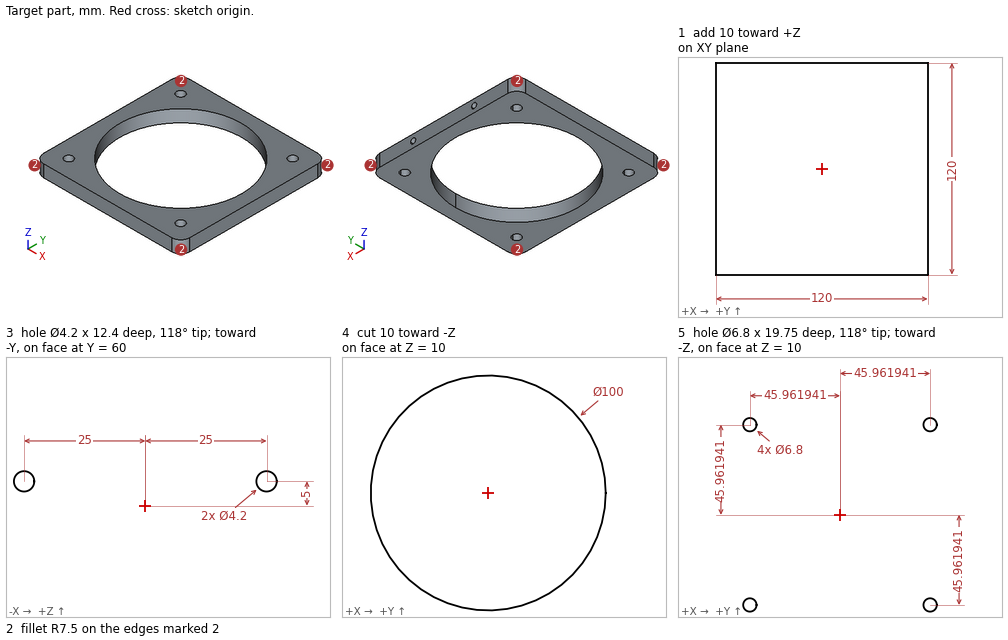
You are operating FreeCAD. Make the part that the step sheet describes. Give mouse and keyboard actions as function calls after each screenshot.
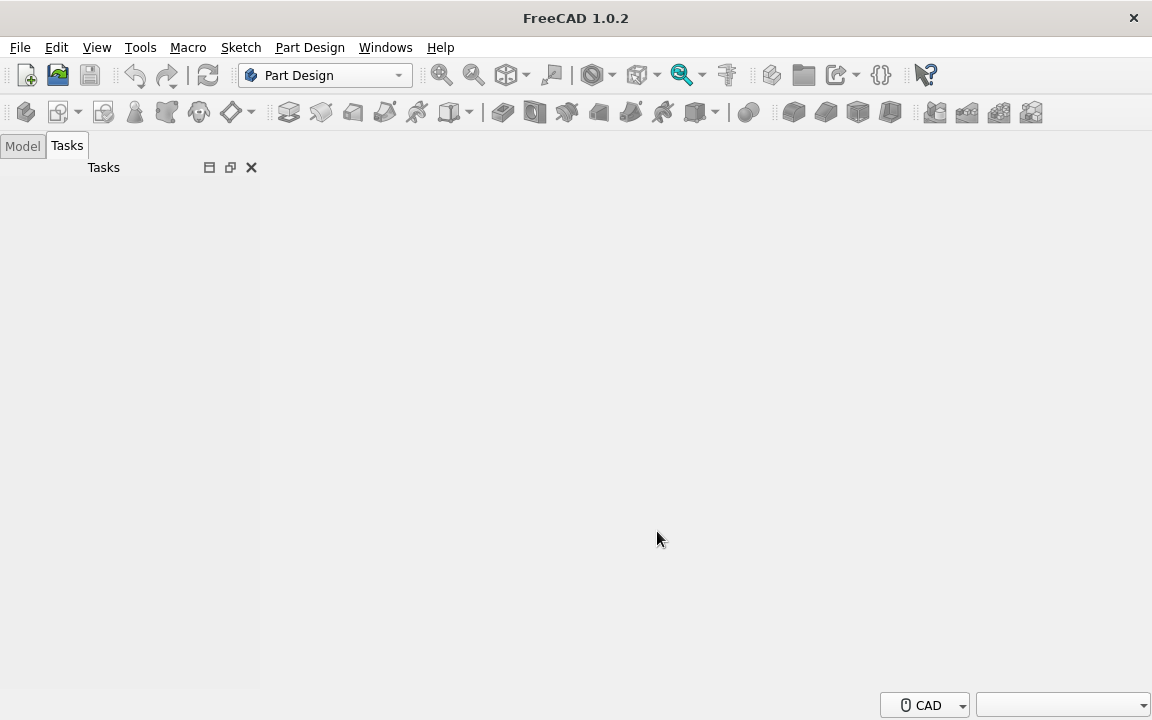
click(26, 76)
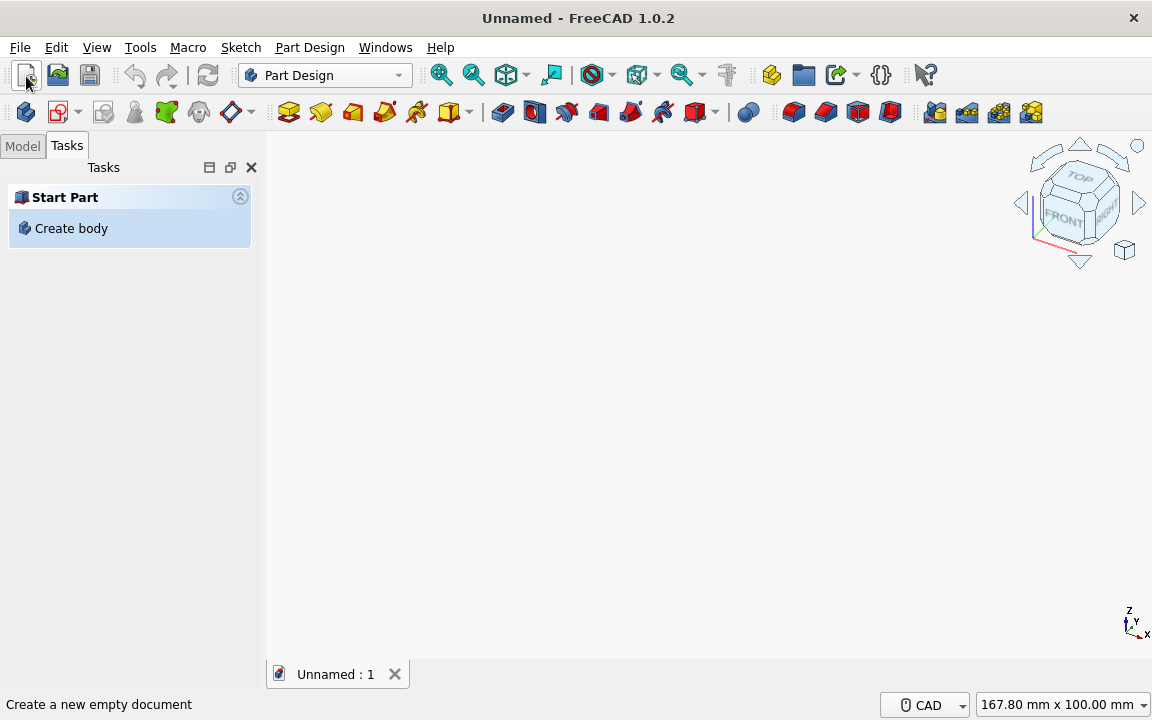
click(58, 112)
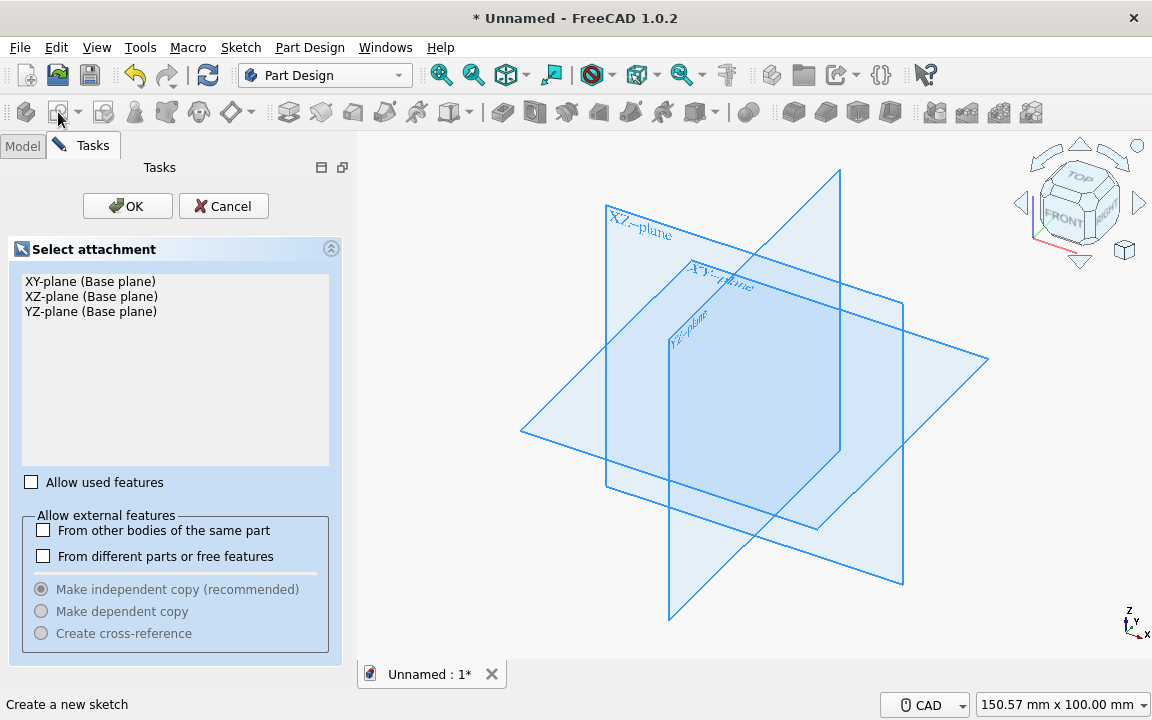
click(82, 282)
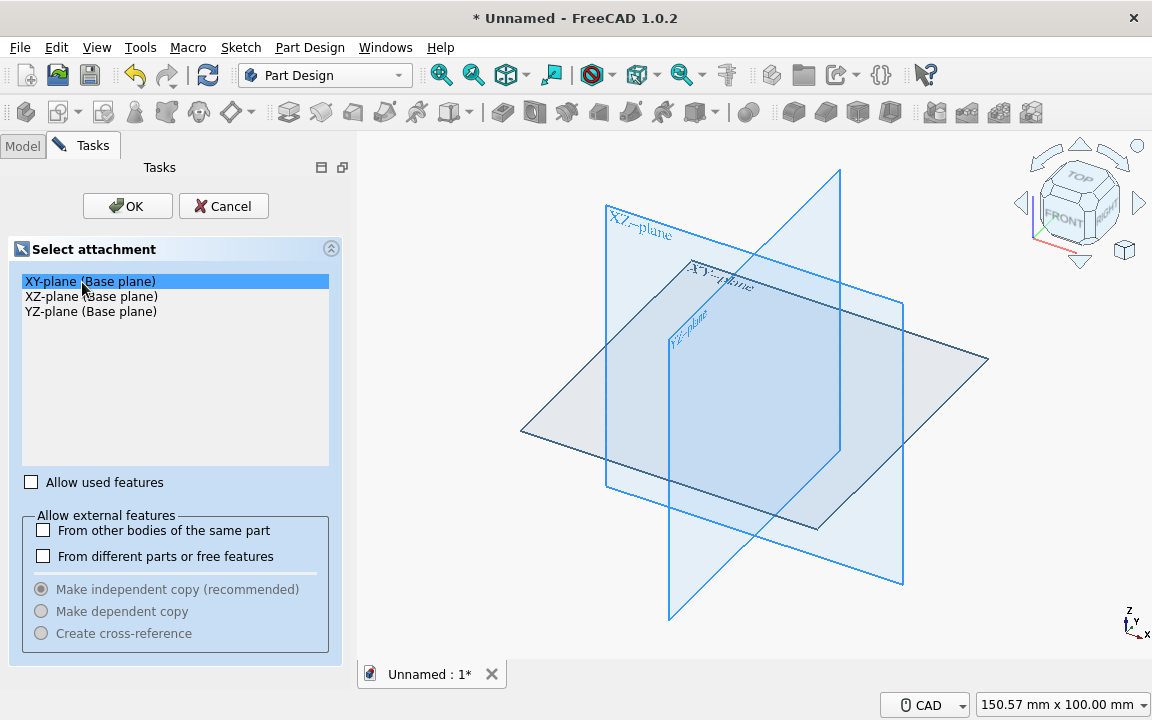
click(128, 206)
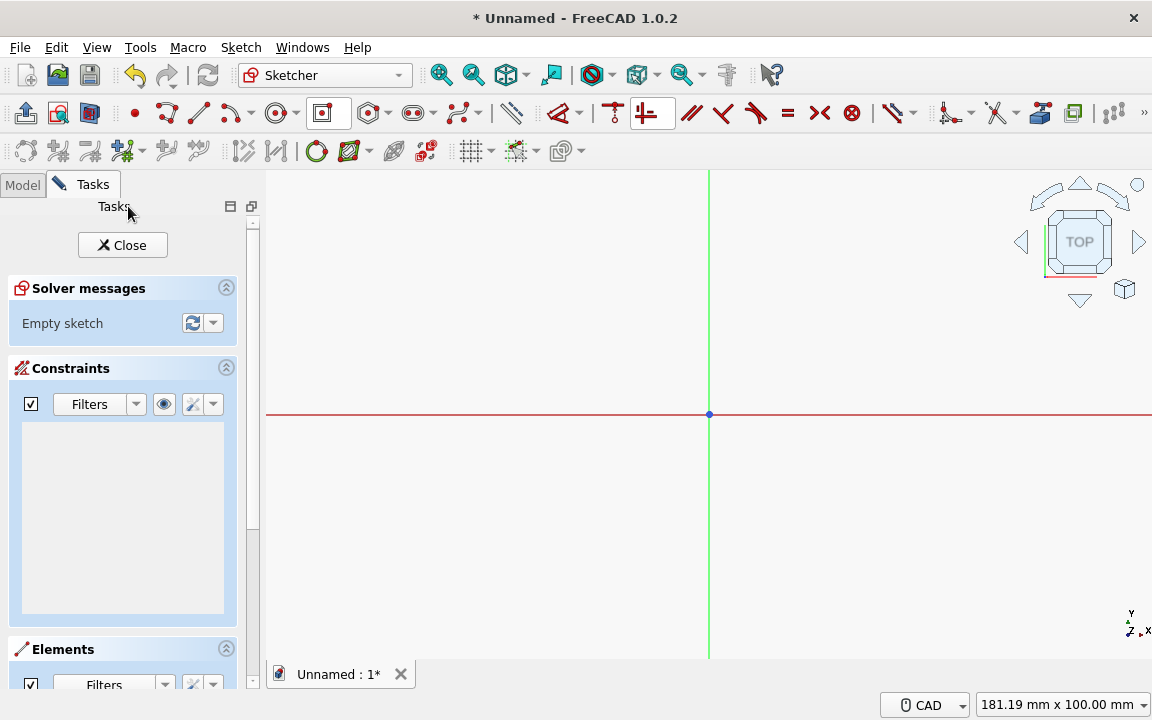
scroll(557, 414, down, 3)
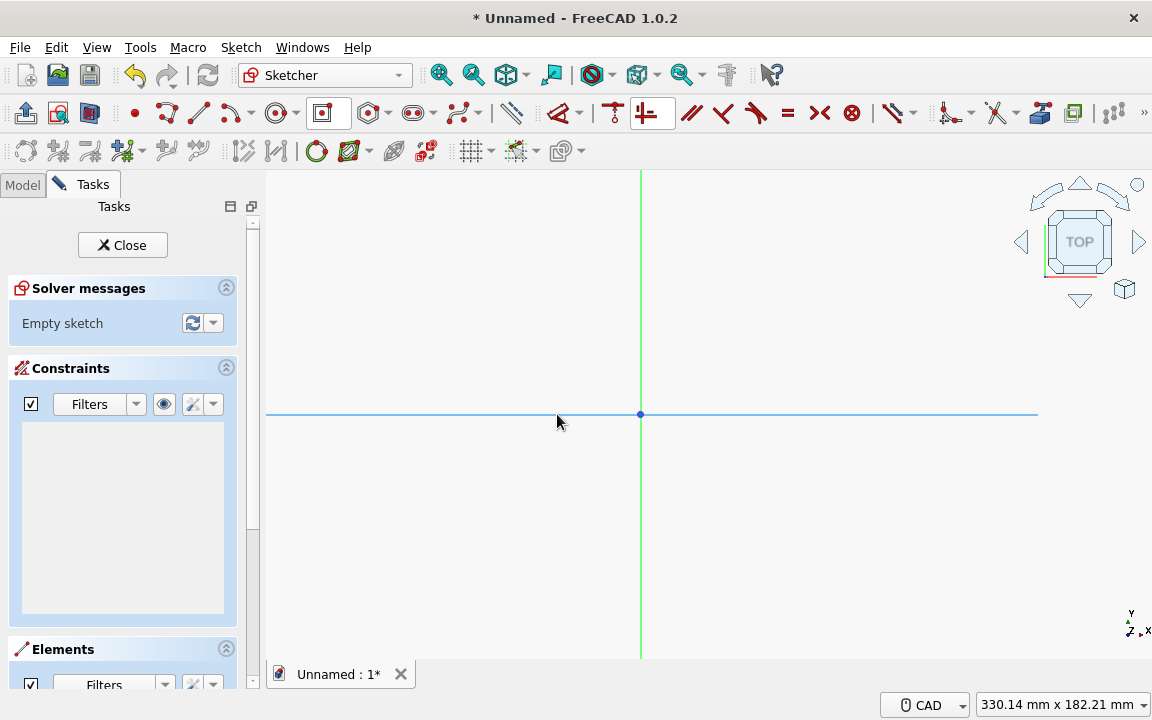
click(322, 114)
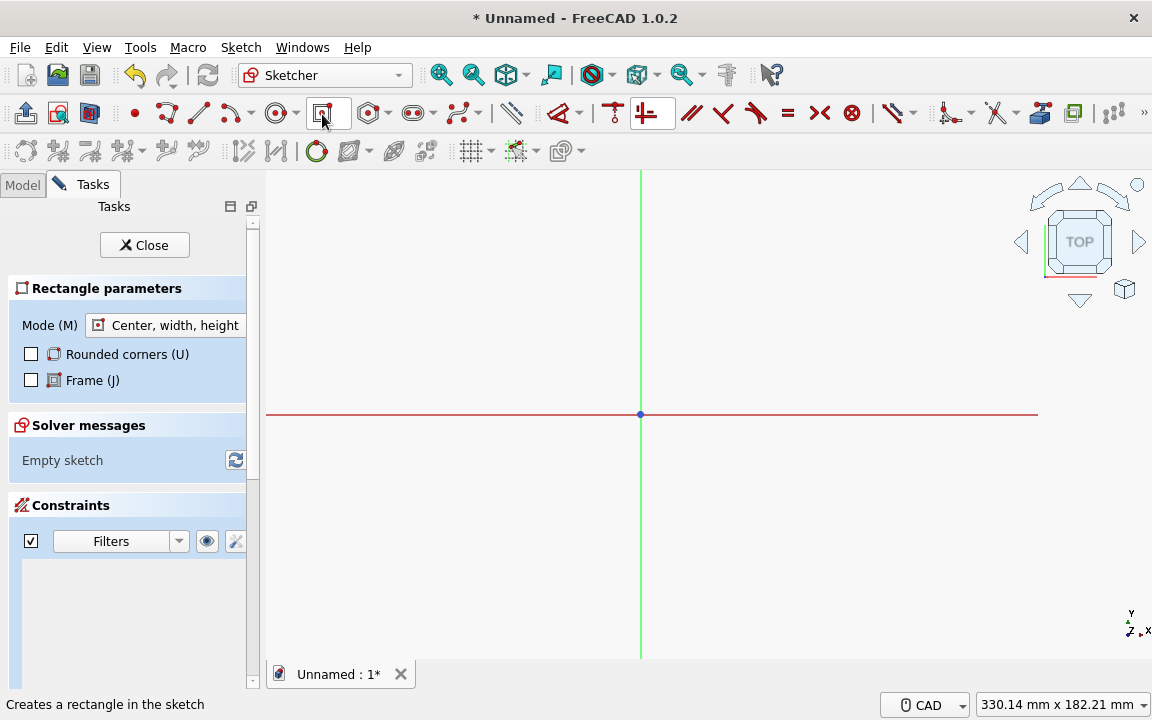
click(641, 414)
click(802, 253)
key(Escape)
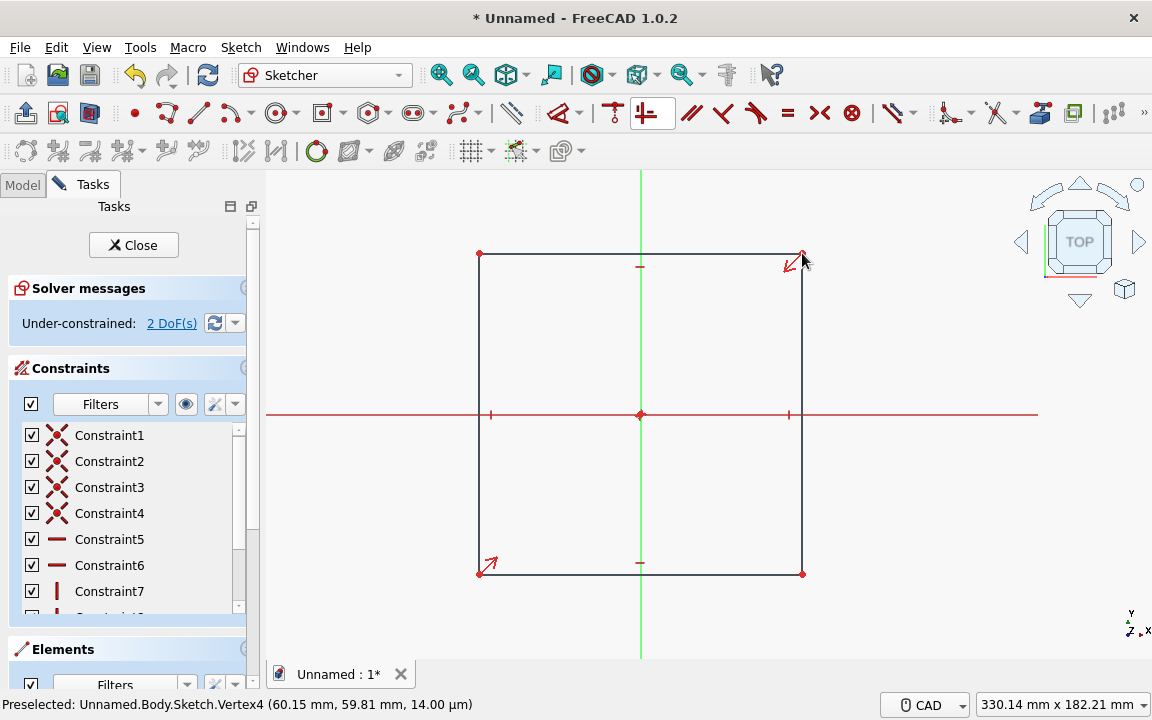
click(558, 114)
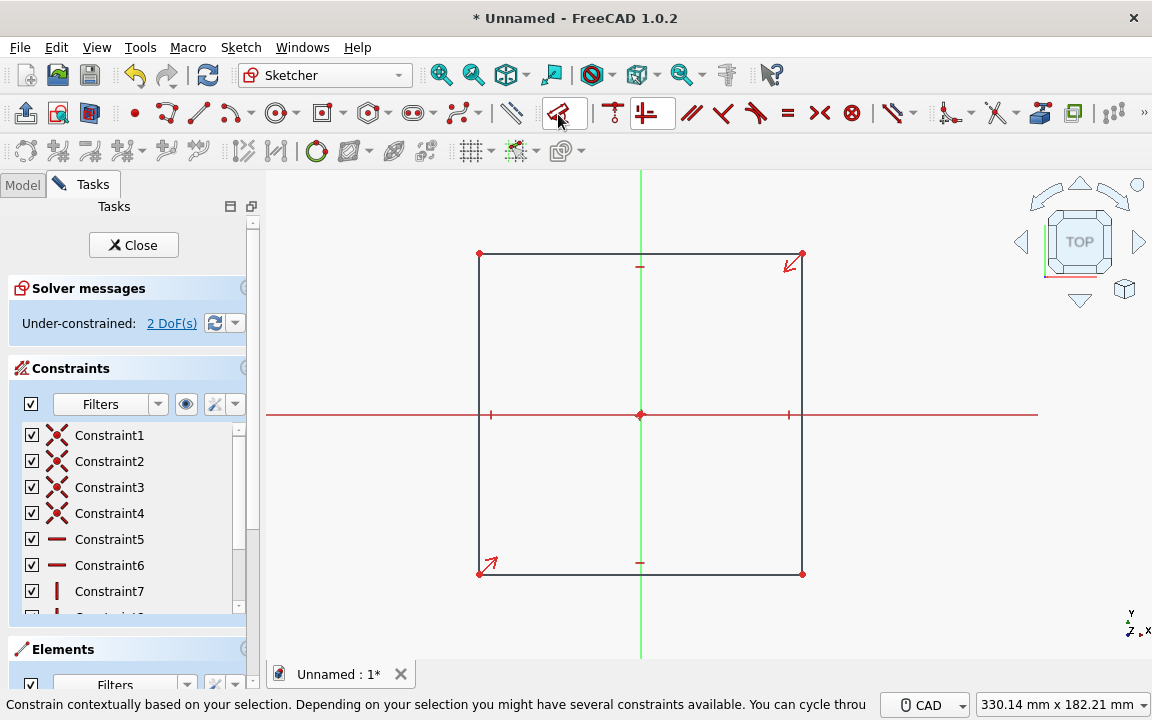
click(576, 575)
click(566, 609)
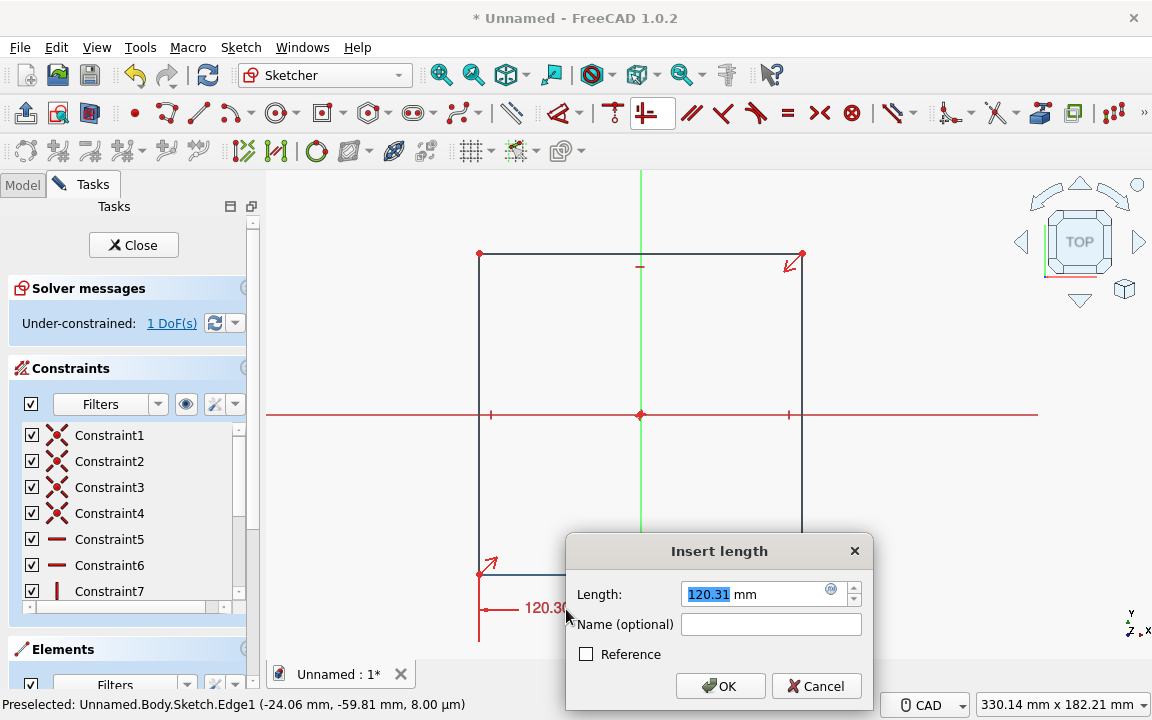
text(120)
key(Return)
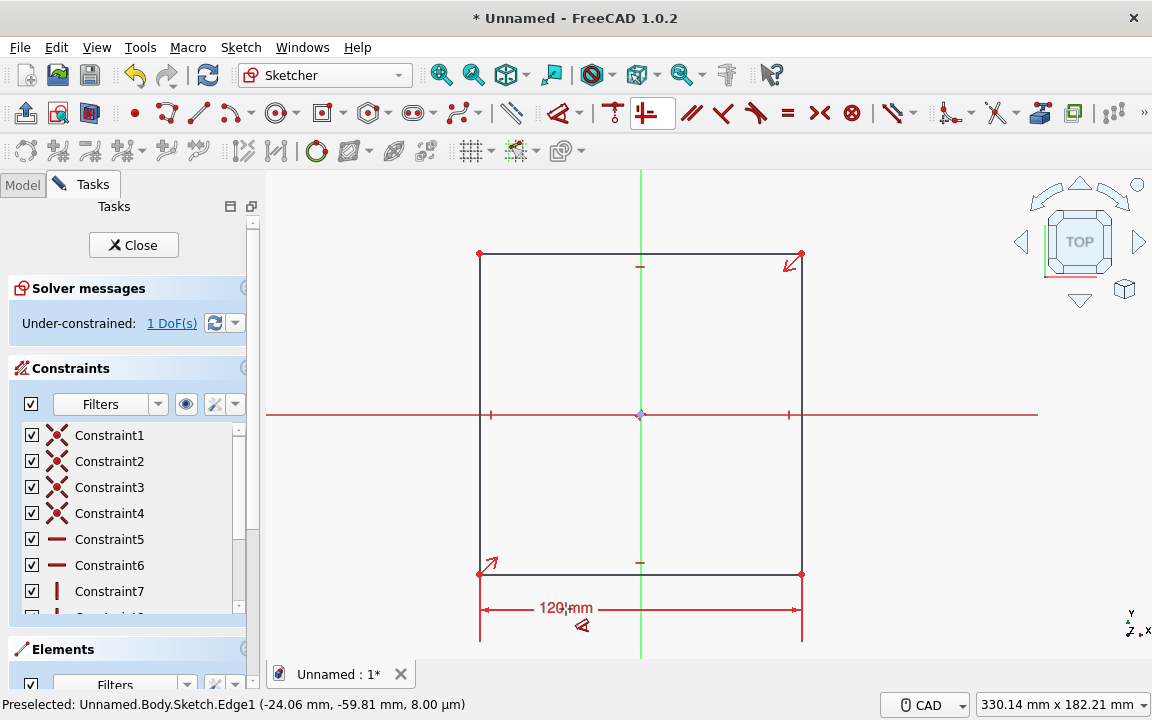
click(802, 479)
click(836, 341)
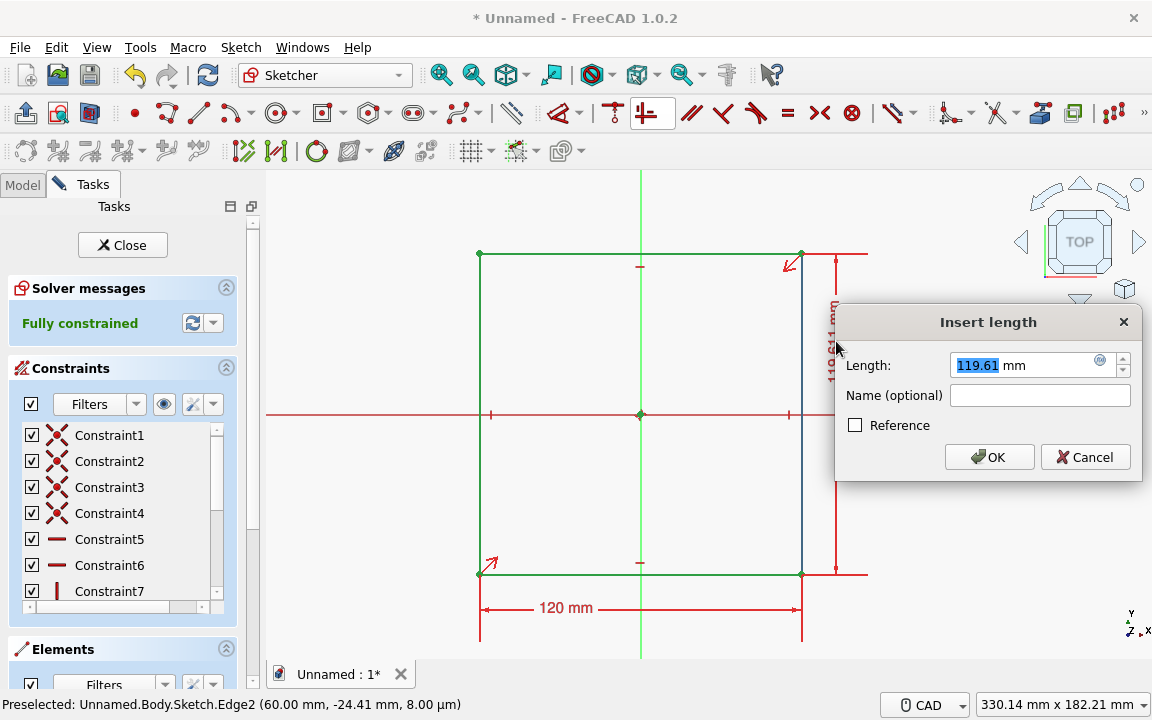
text(120)
key(Return)
key(Escape)